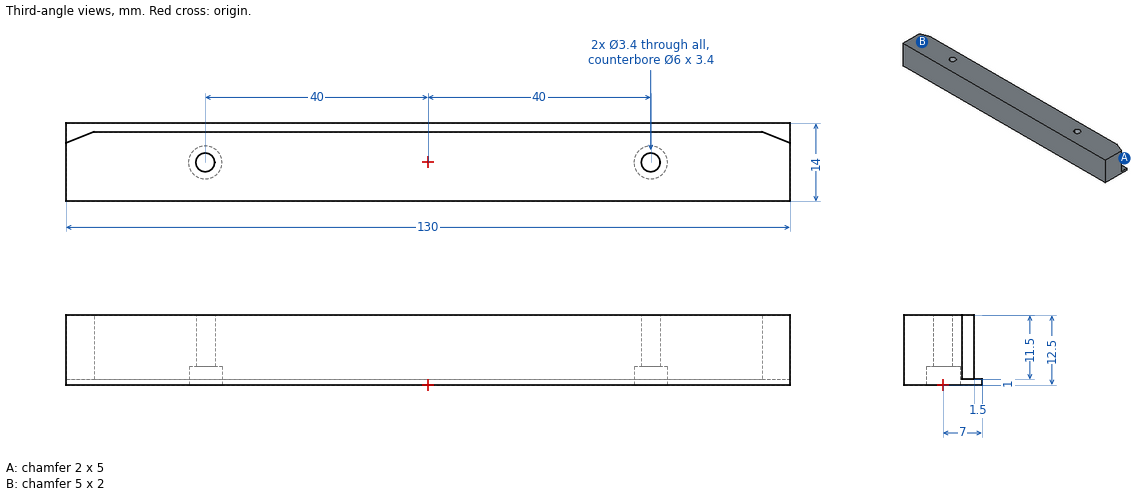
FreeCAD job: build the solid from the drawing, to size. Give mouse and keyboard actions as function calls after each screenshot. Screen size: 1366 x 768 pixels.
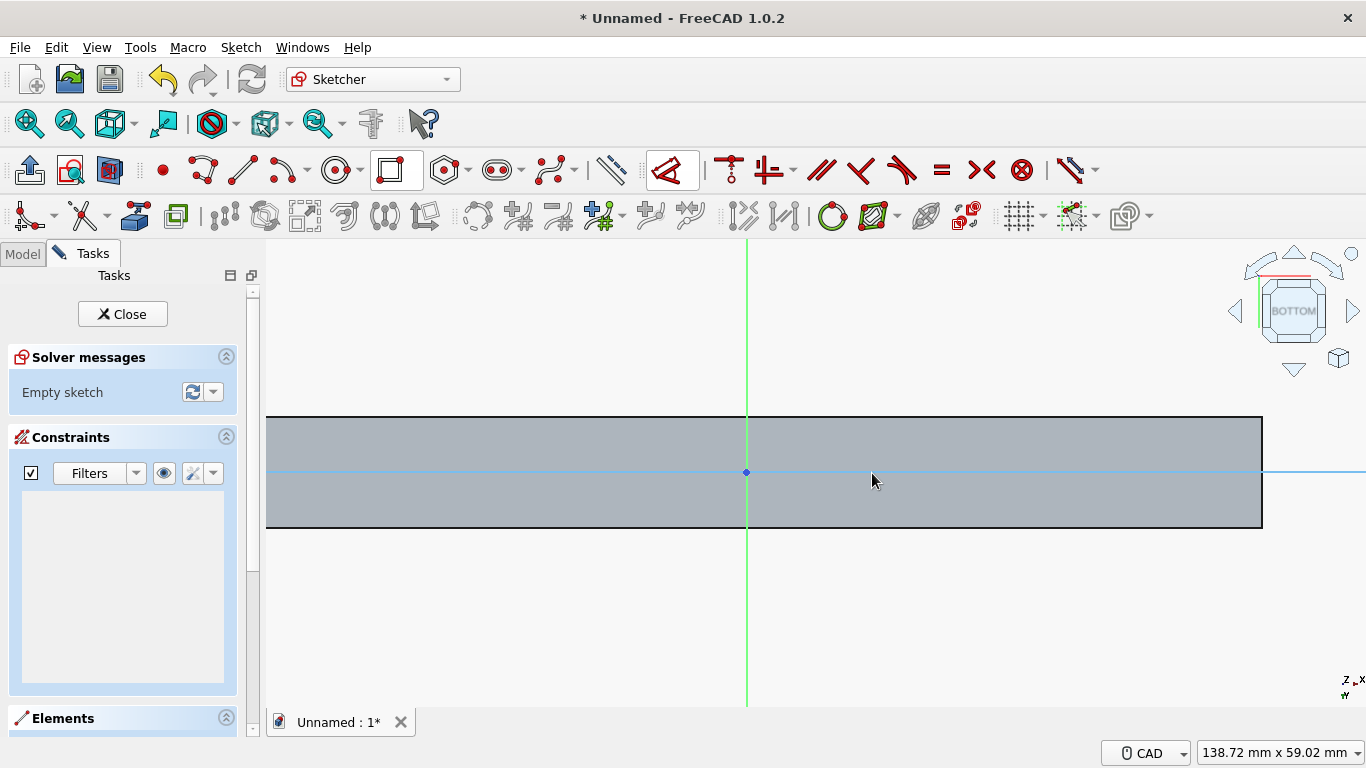
click(336, 170)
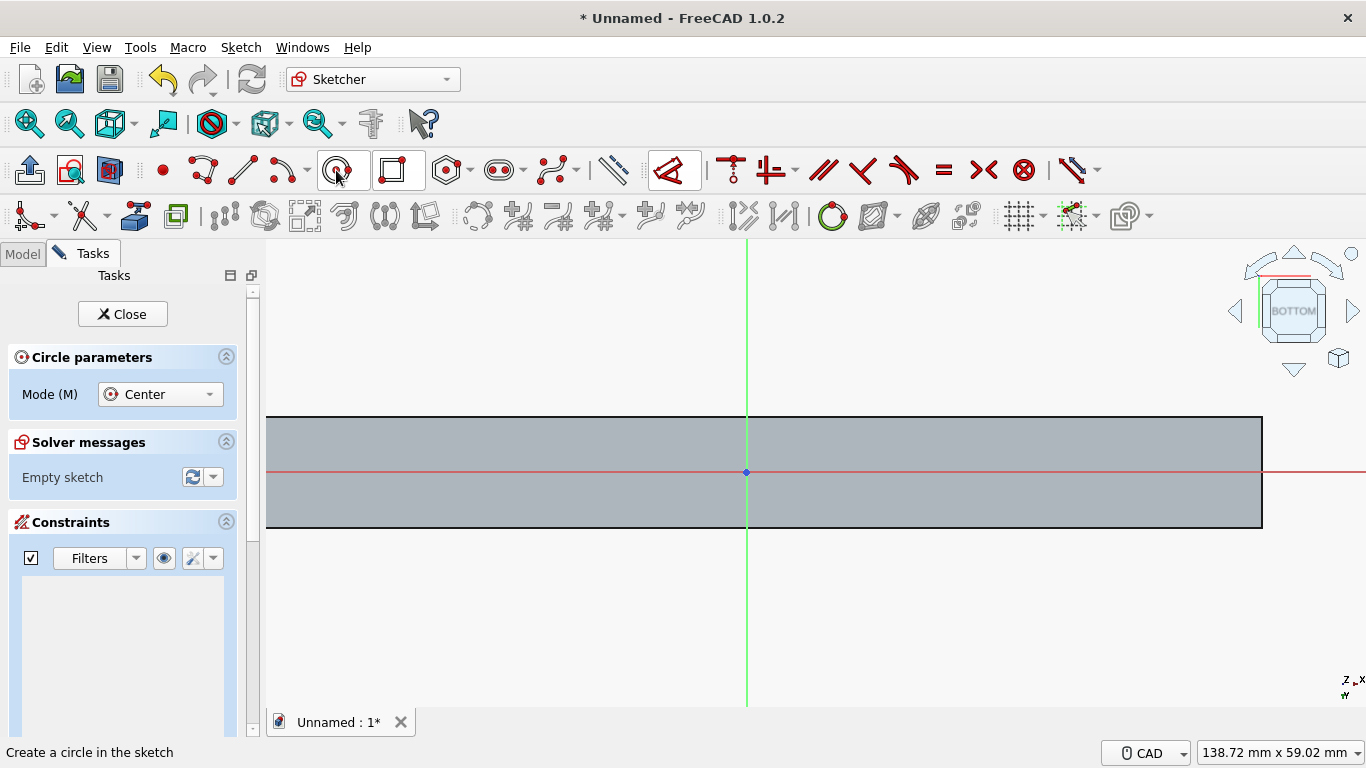
scroll(1064, 472, up, 3)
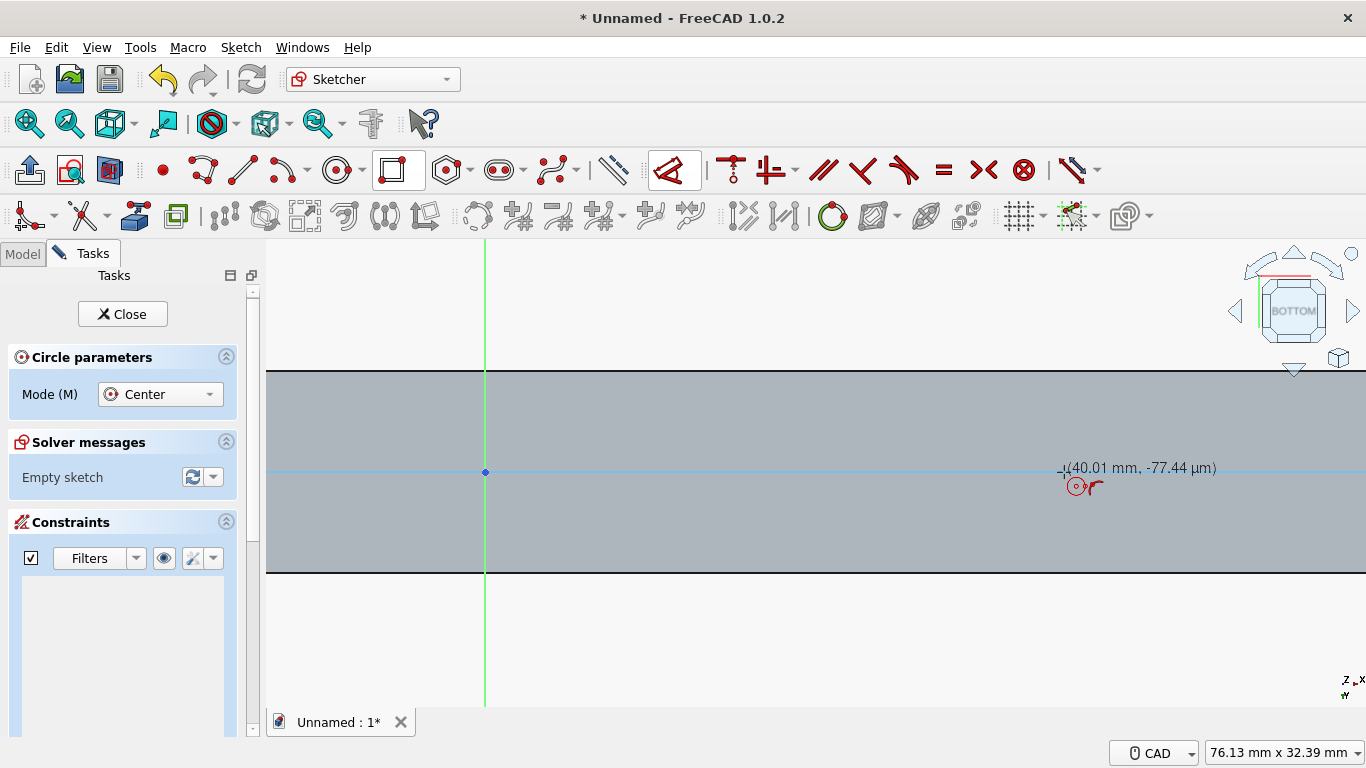
click(1063, 472)
click(1081, 455)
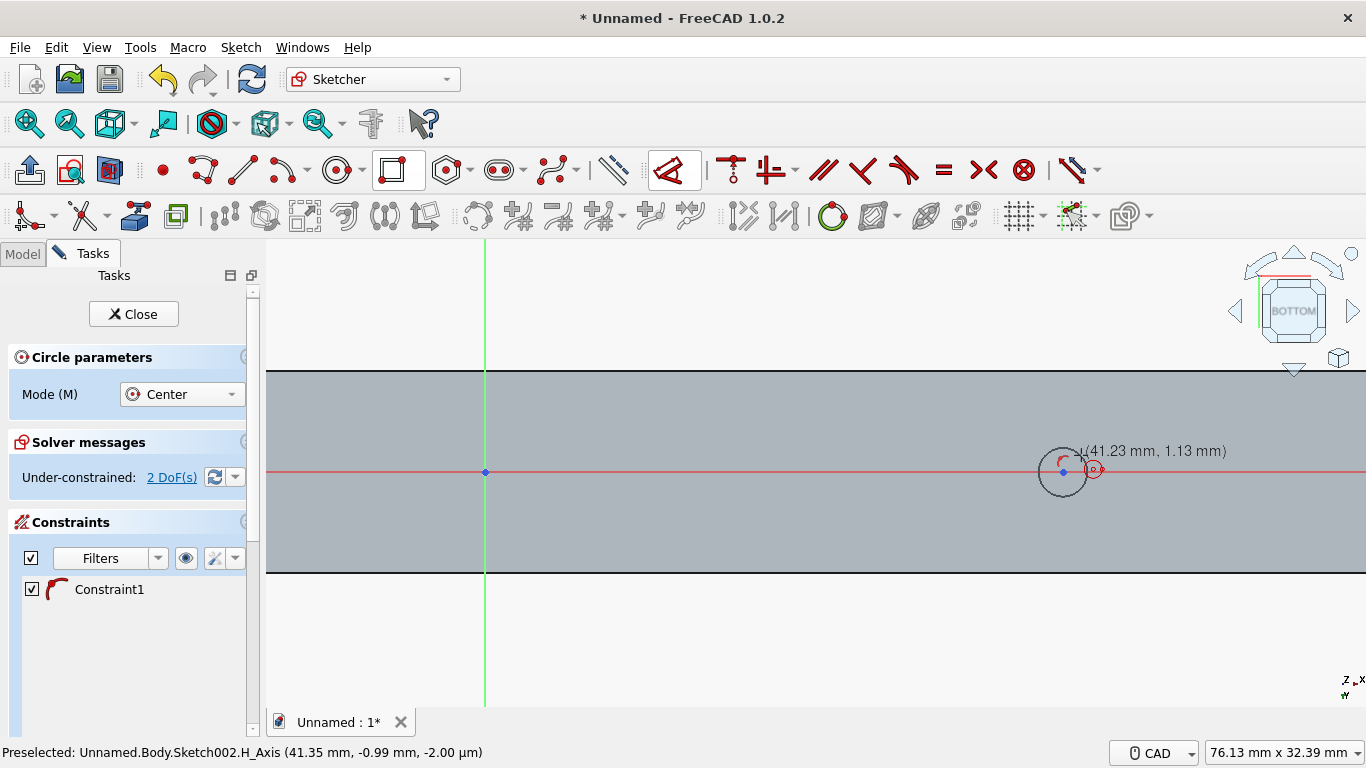
scroll(1067, 474, down, 3)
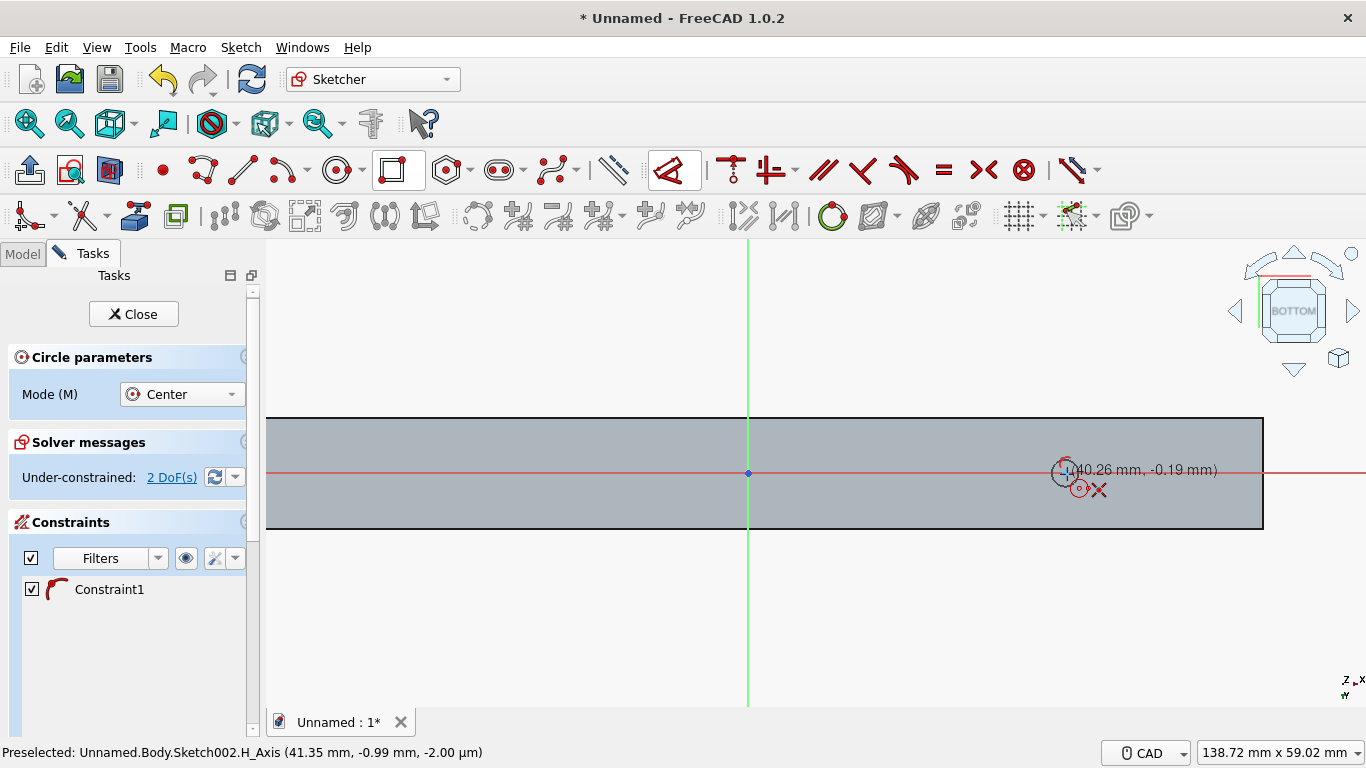
scroll(431, 473, up, 3)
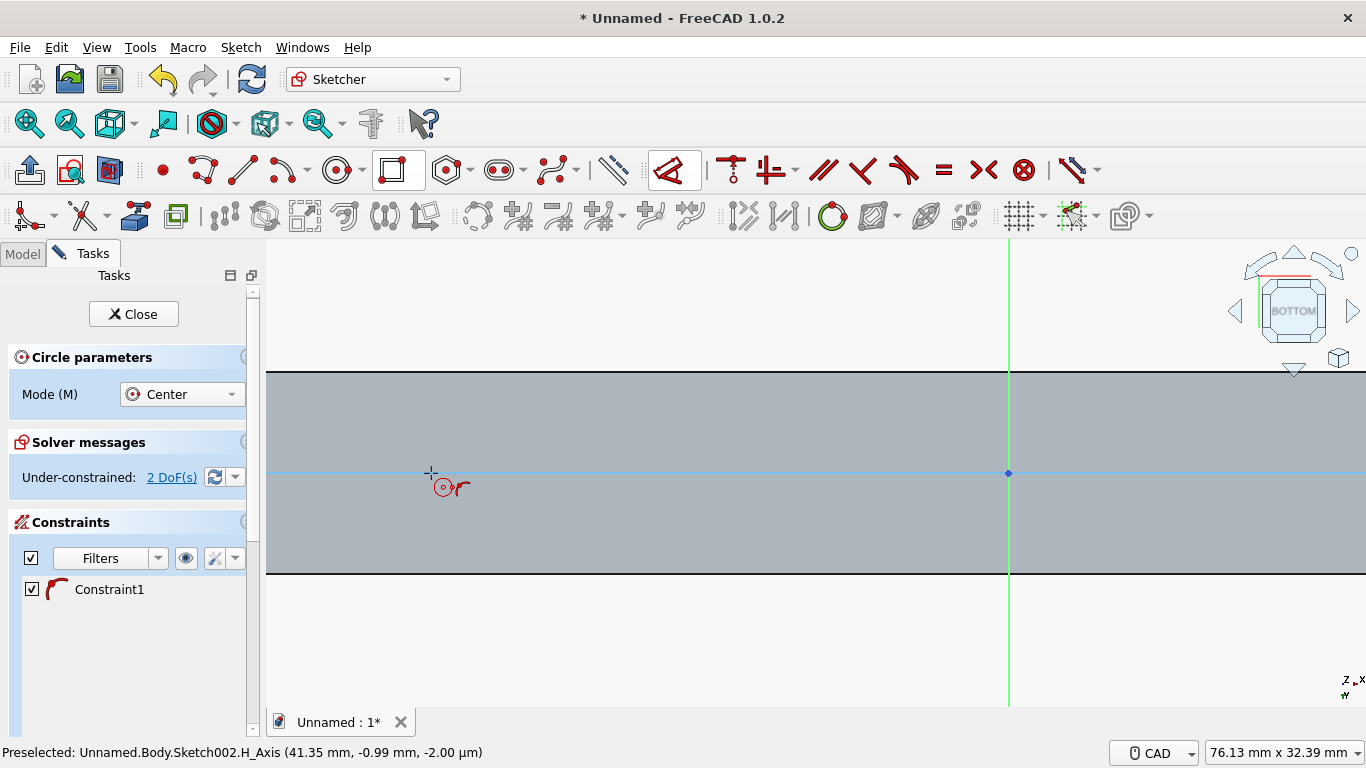
click(431, 473)
click(448, 456)
key(Escape)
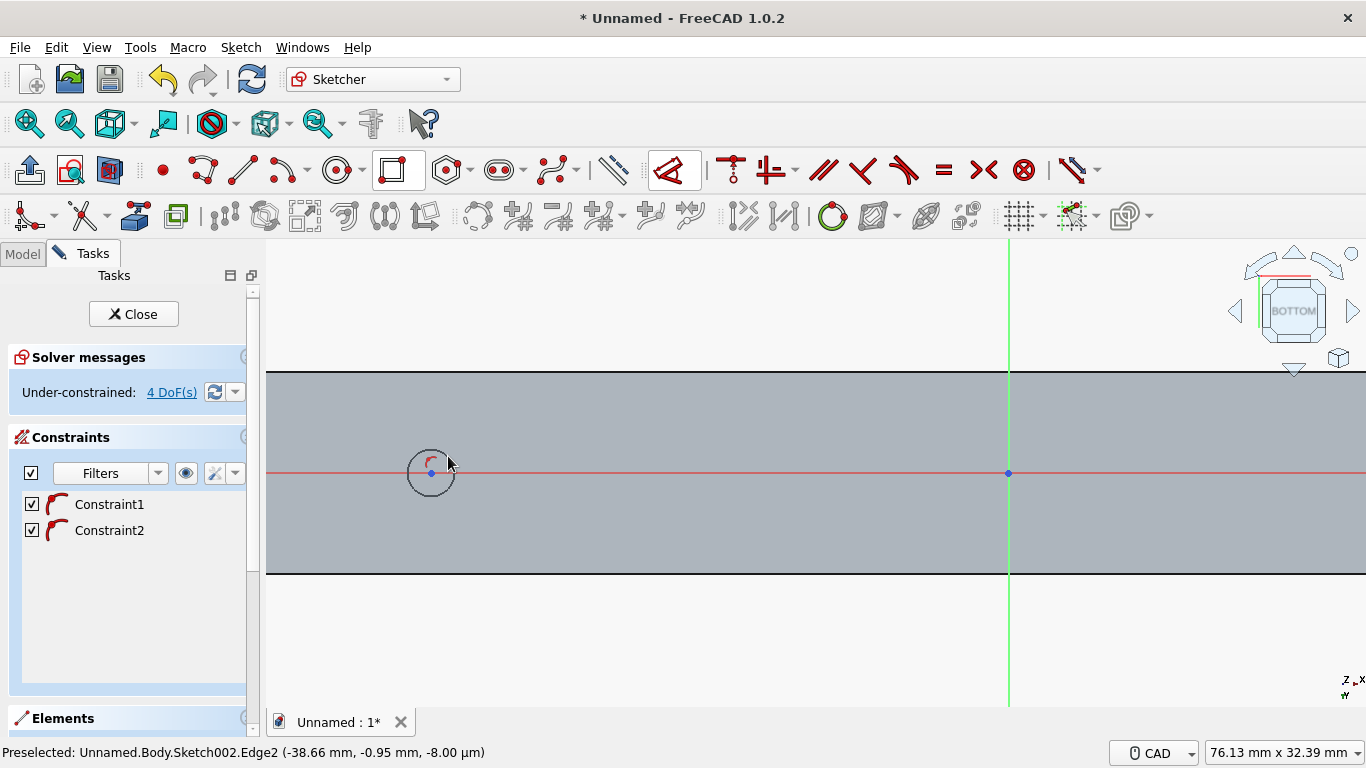
scroll(430, 473, down, 3)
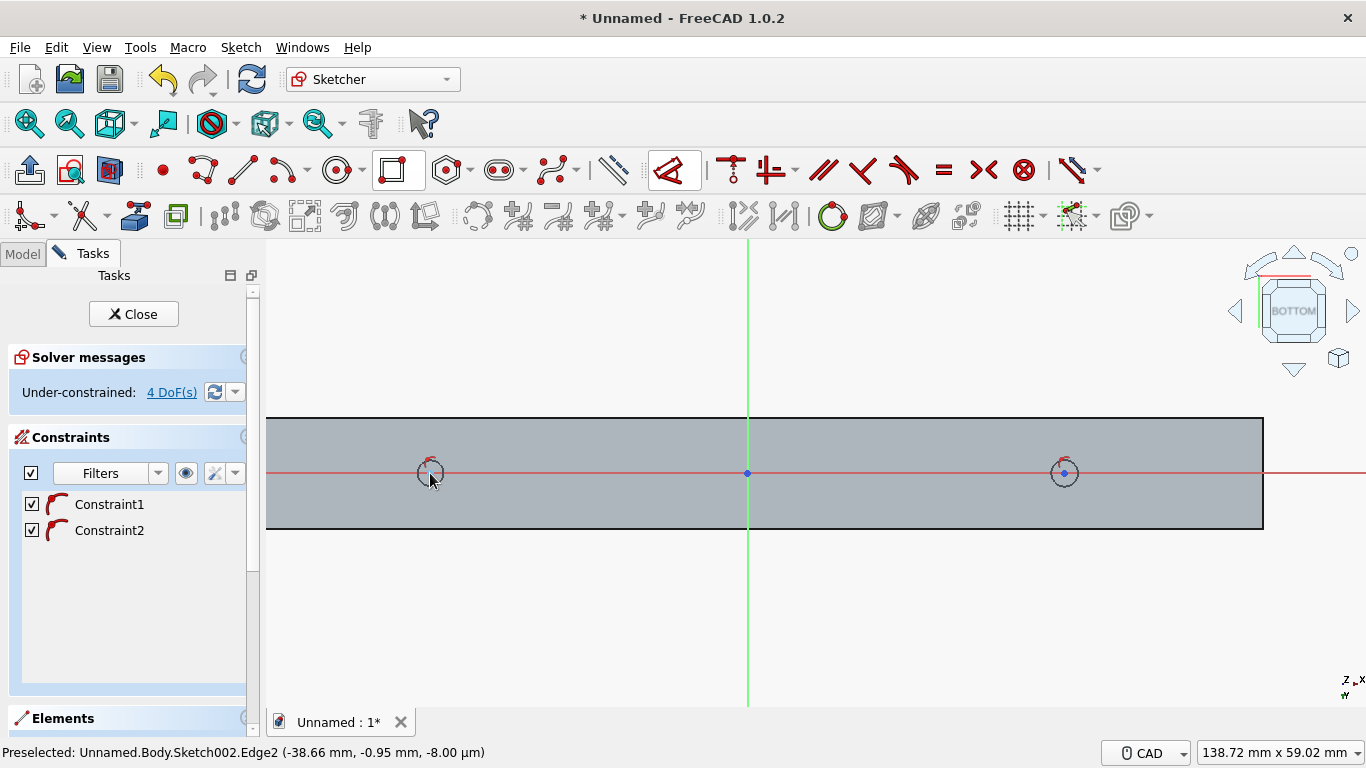
scroll(1074, 464, up, 2)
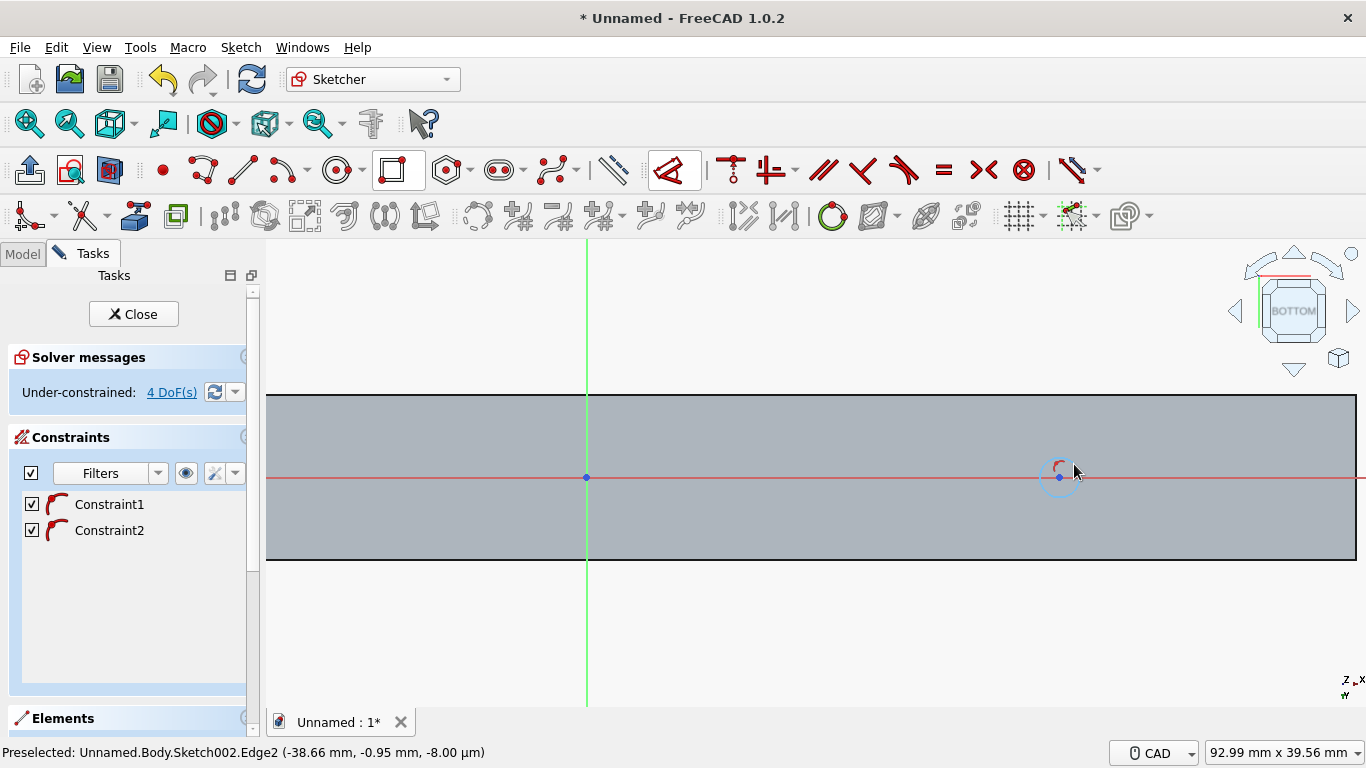
click(1074, 464)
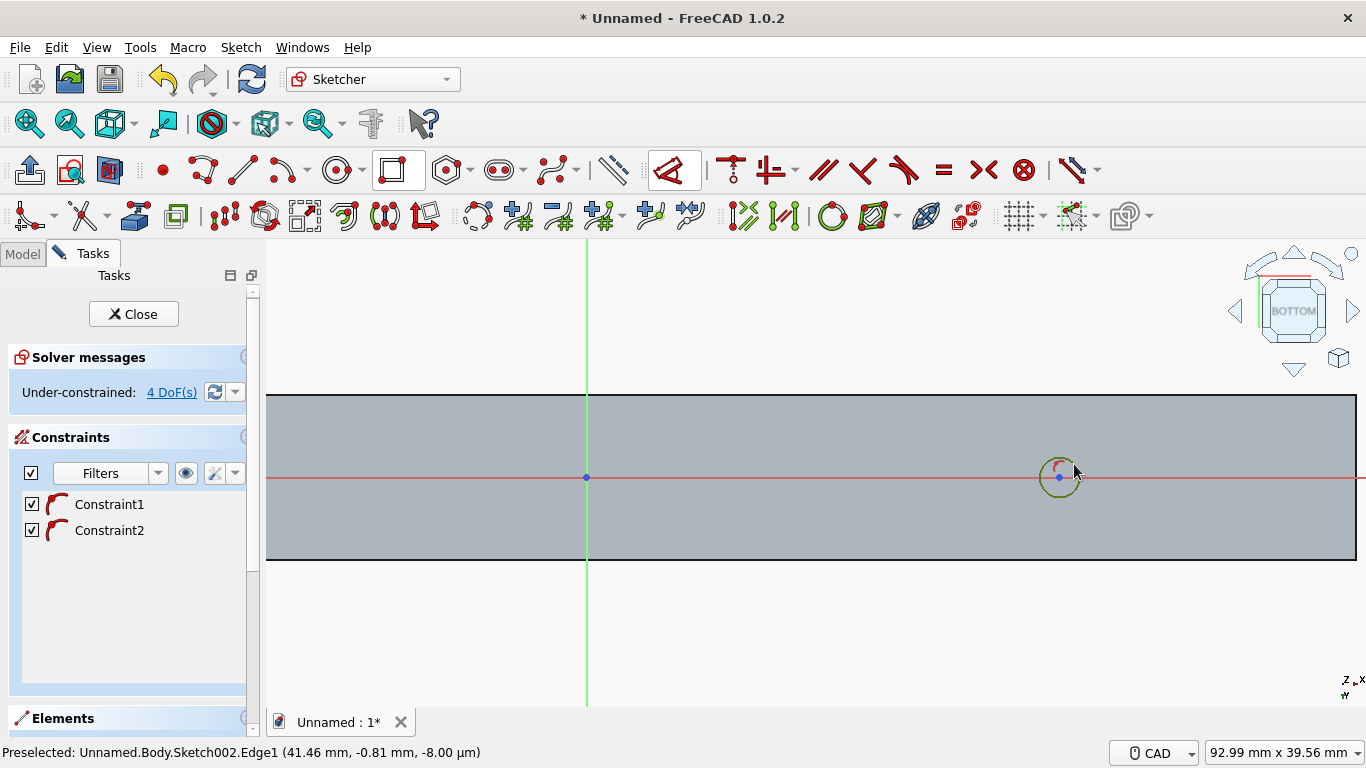
scroll(1074, 464, down, 2)